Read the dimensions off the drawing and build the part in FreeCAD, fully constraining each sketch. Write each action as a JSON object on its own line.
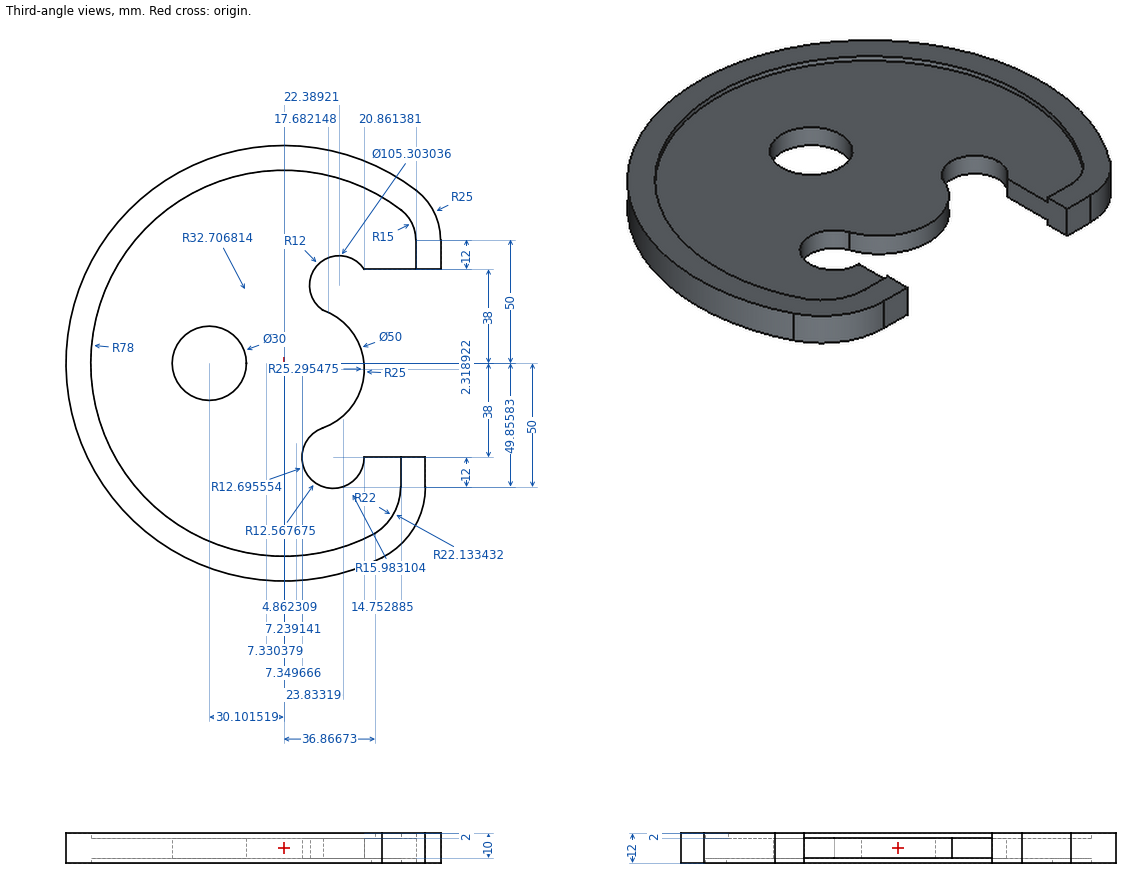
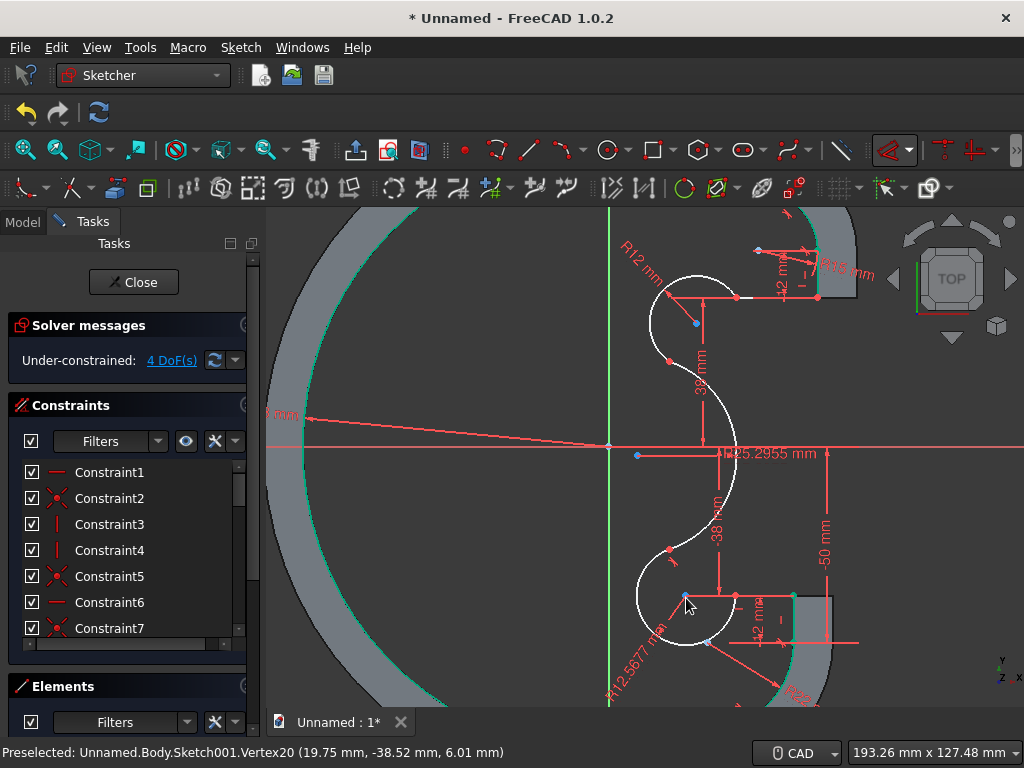
{"action": "left_click", "coordinate": [761, 298]}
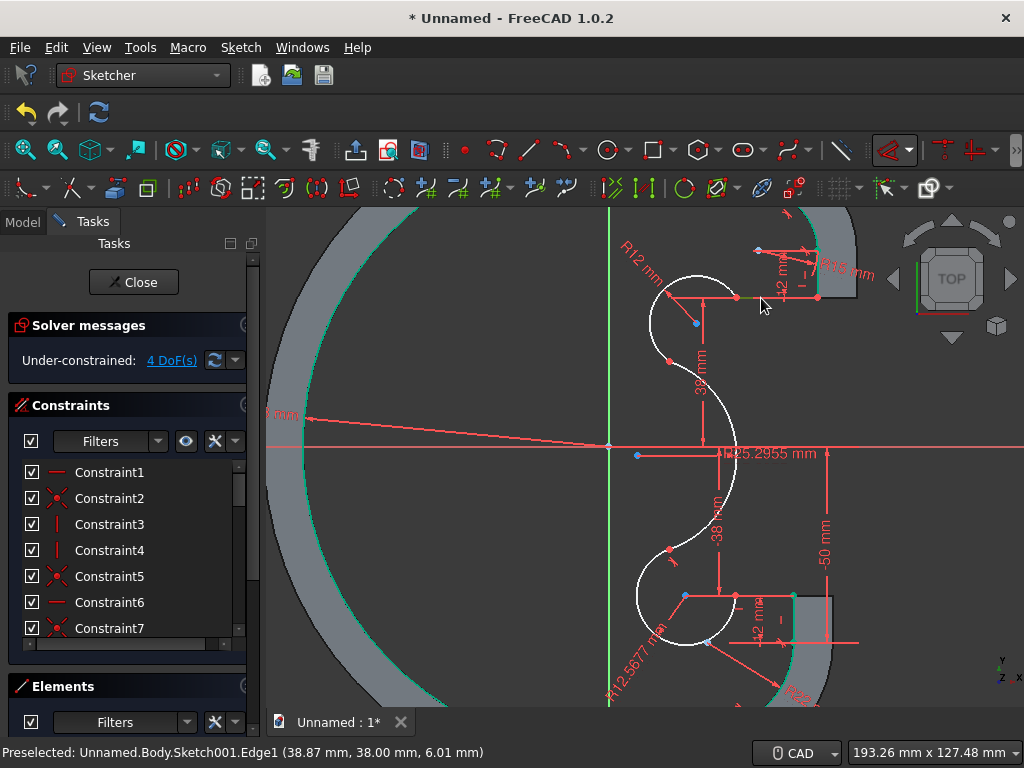
{"action": "key", "text": "l"}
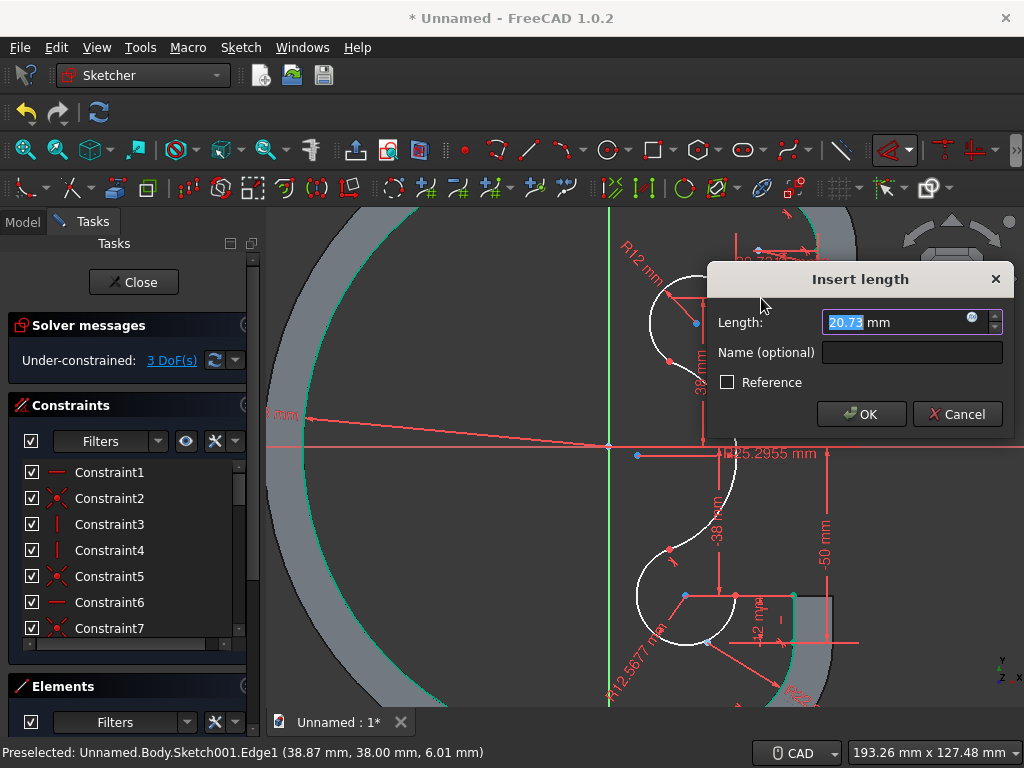
{"action": "type", "text": "20.861381"}
{"action": "key", "text": "Return"}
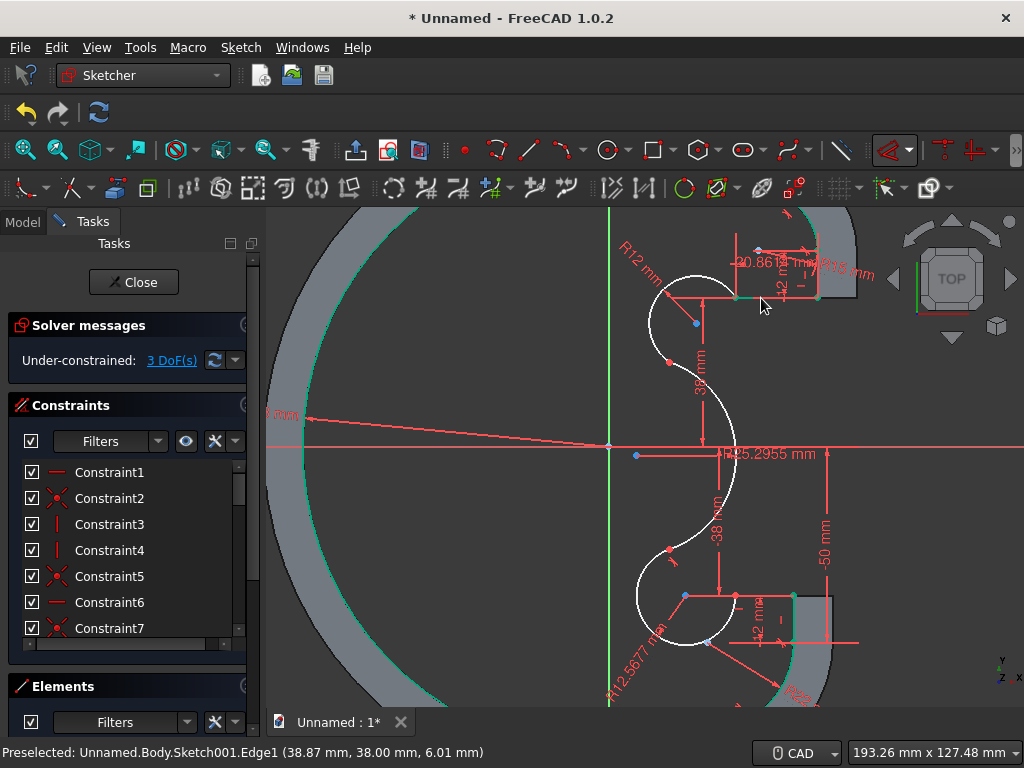
{"action": "left_click", "coordinate": [776, 596]}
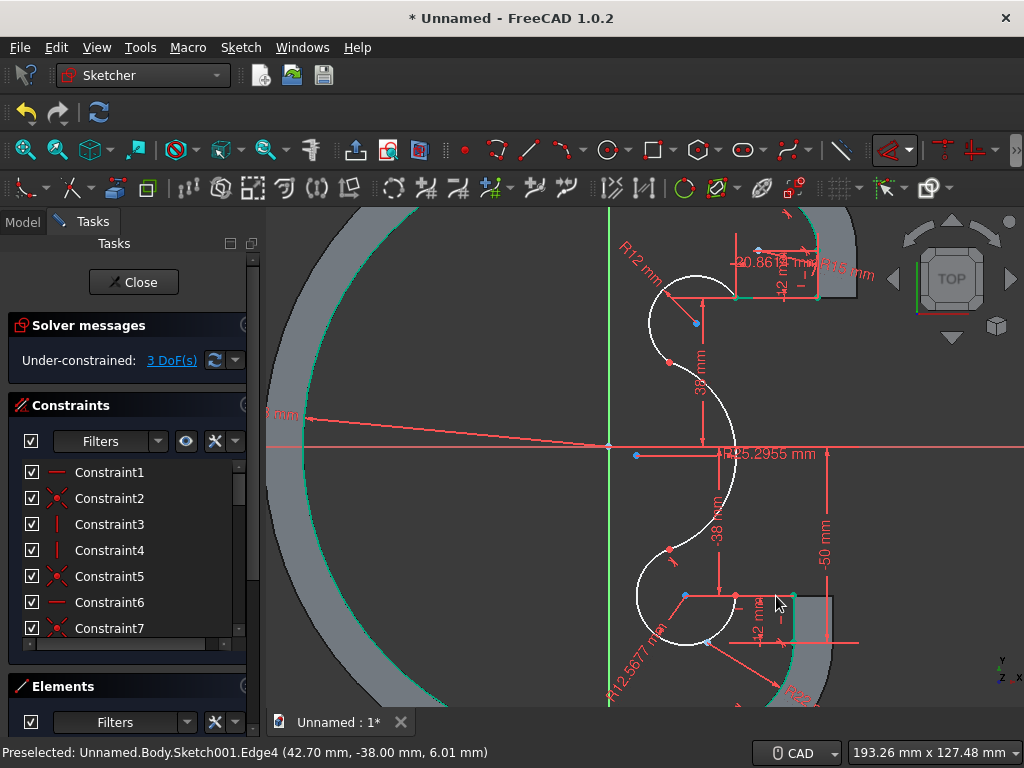
{"action": "key", "text": "l"}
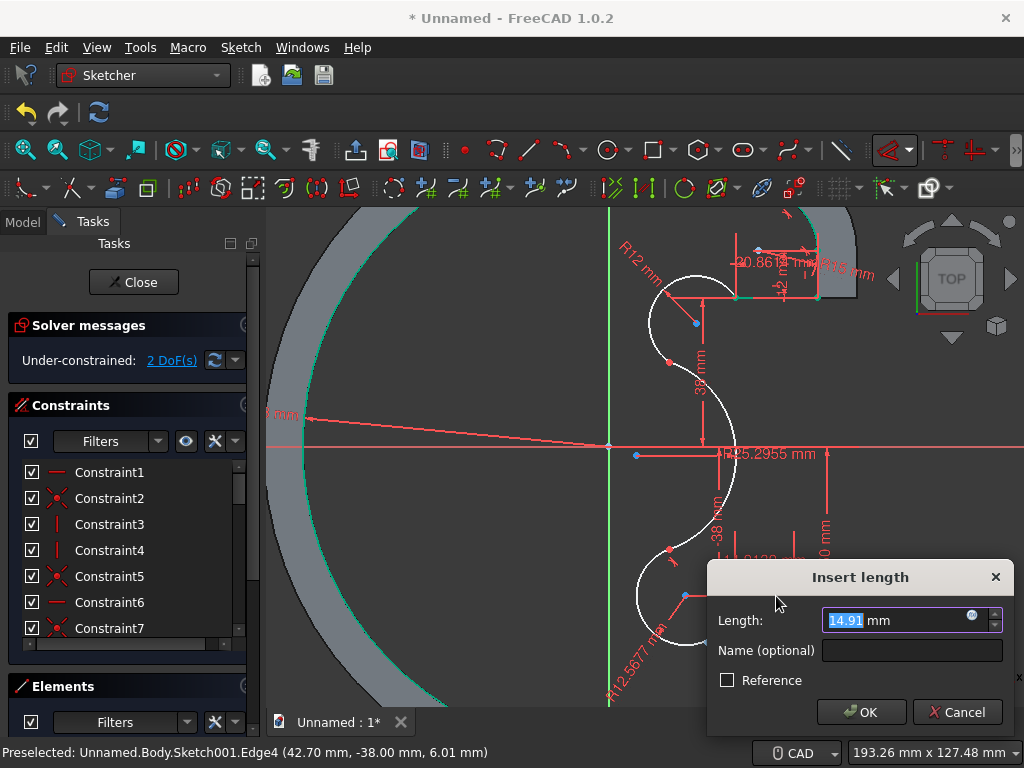
{"action": "type", "text": "14.752885"}
{"action": "key", "text": "Return"}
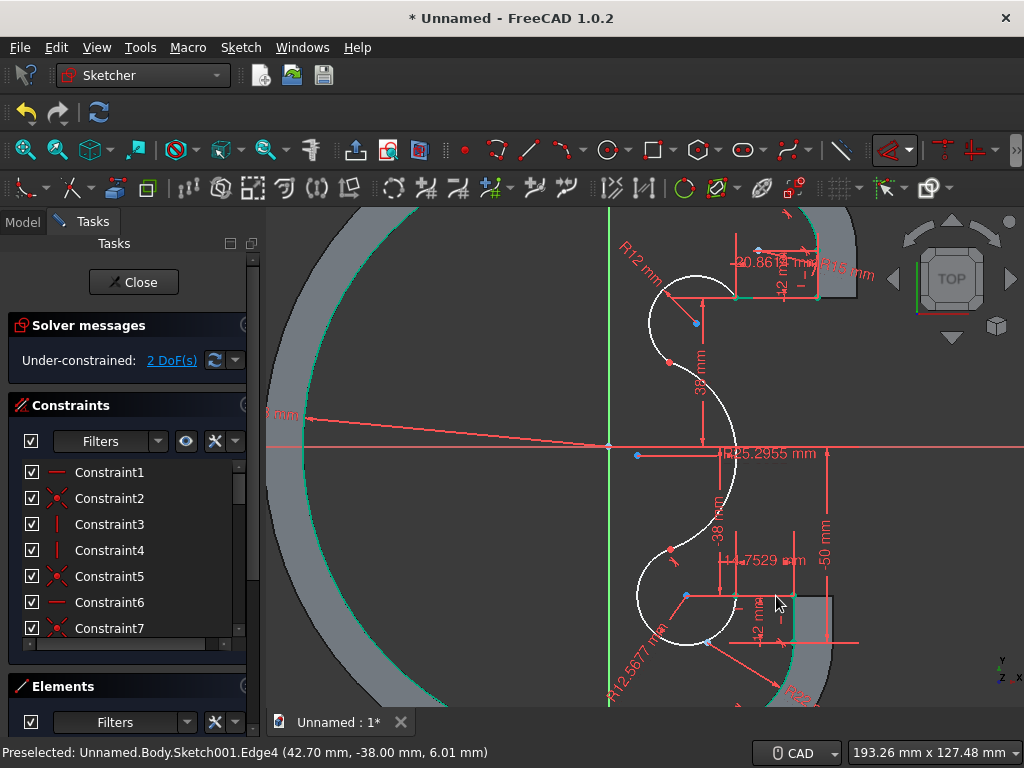
{"action": "scroll", "coordinate": [637, 456], "scroll_direction": "up", "scroll_amount": 2}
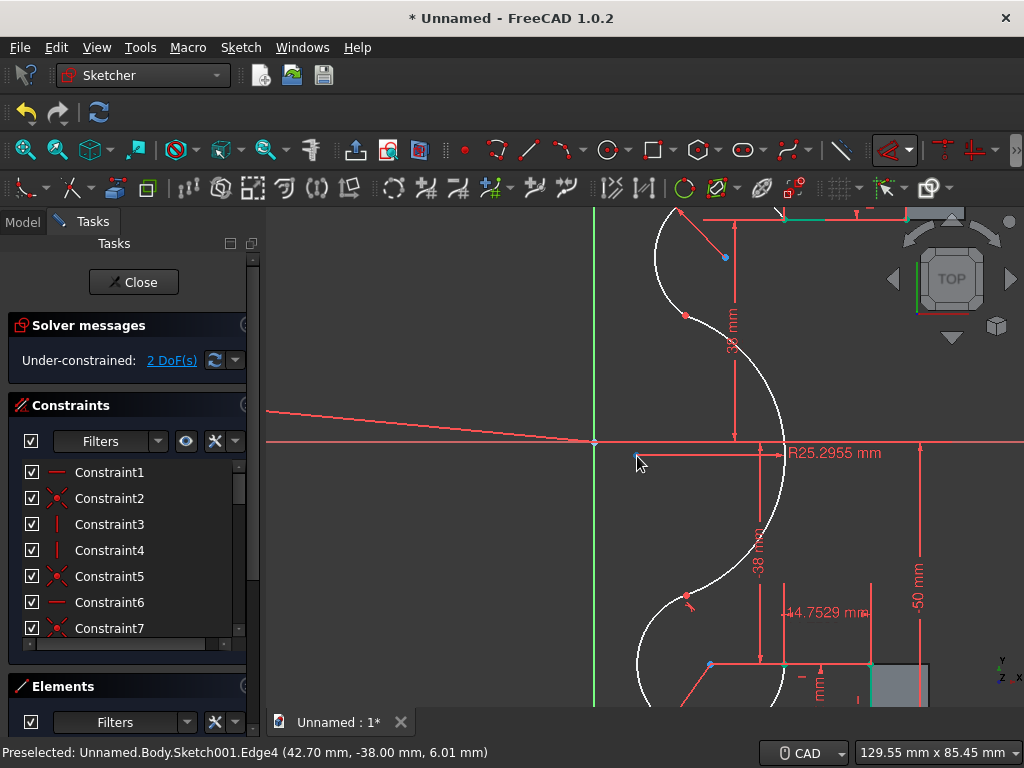
{"action": "left_click", "coordinate": [637, 455]}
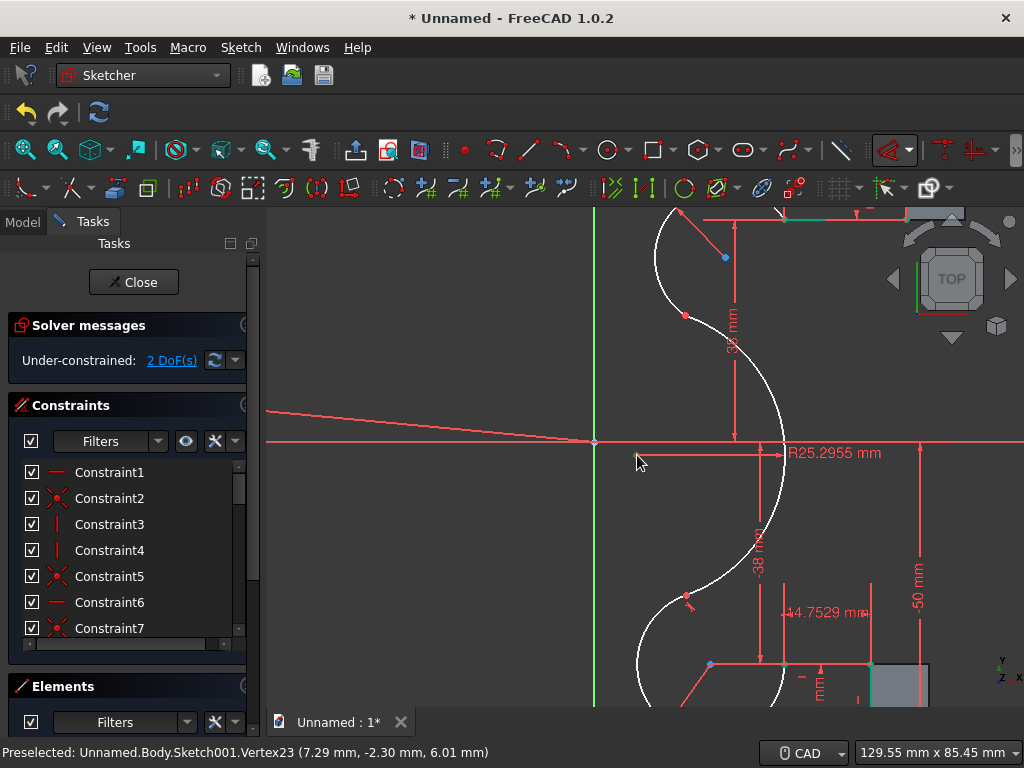
{"action": "key", "text": "l"}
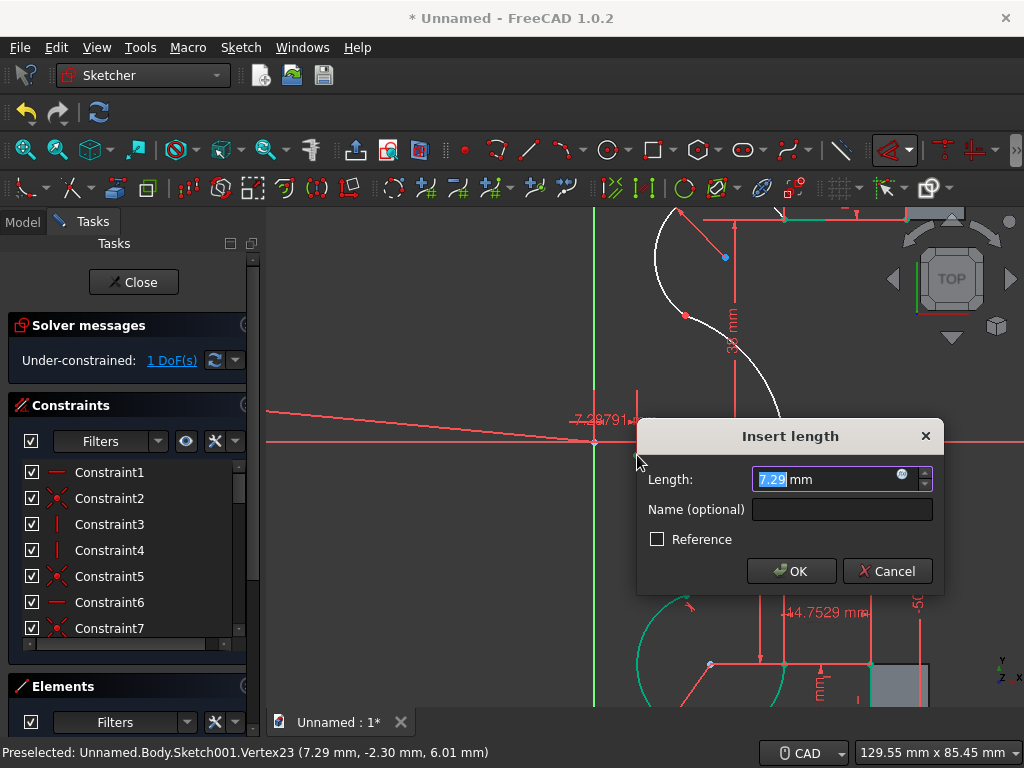
{"action": "type", "text": "7.239141"}
{"action": "key", "text": "Return"}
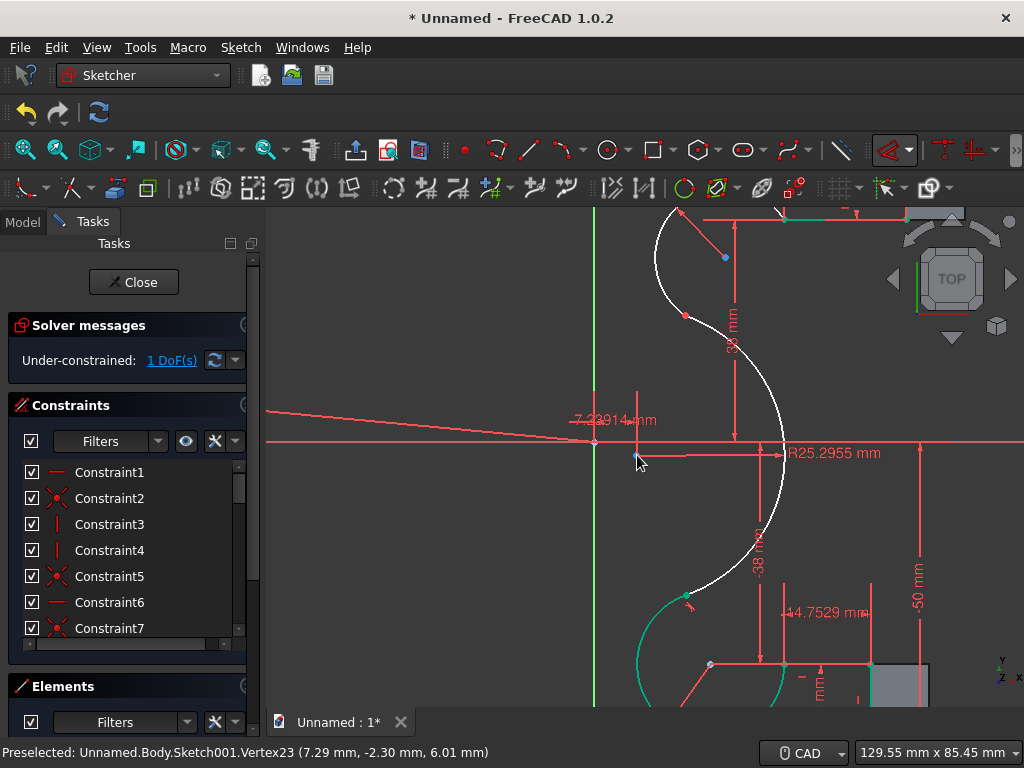
{"action": "left_click", "coordinate": [725, 258]}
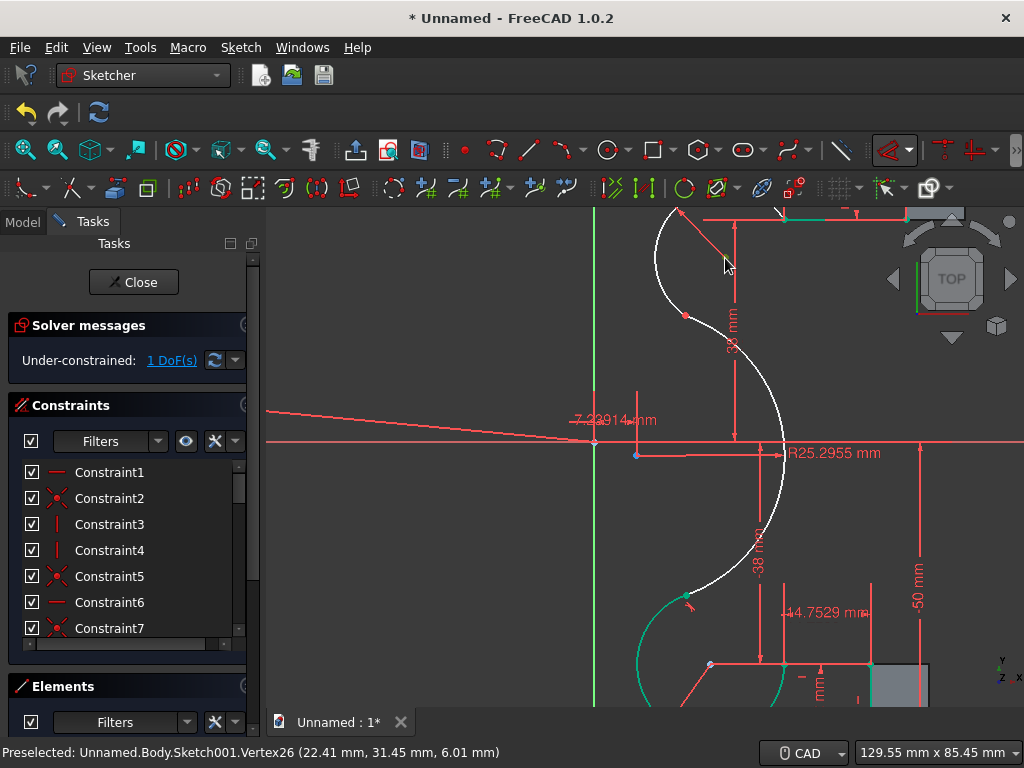
{"action": "key", "text": "l"}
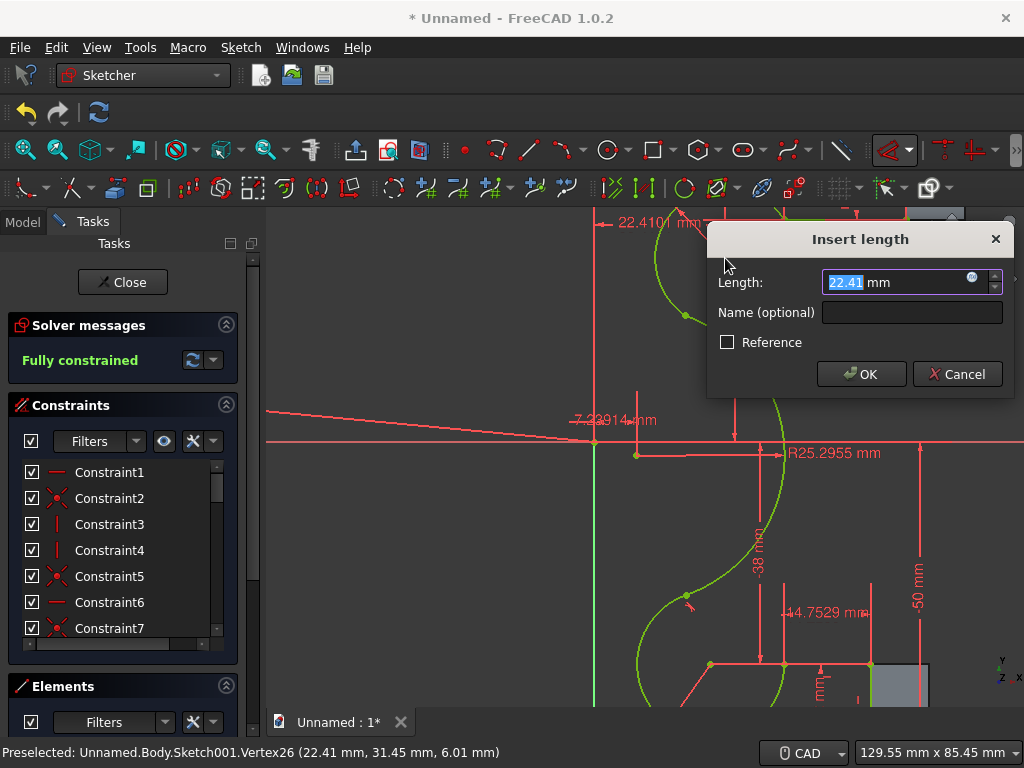
{"action": "type", "text": "22.38921"}
{"action": "key", "text": "Return"}